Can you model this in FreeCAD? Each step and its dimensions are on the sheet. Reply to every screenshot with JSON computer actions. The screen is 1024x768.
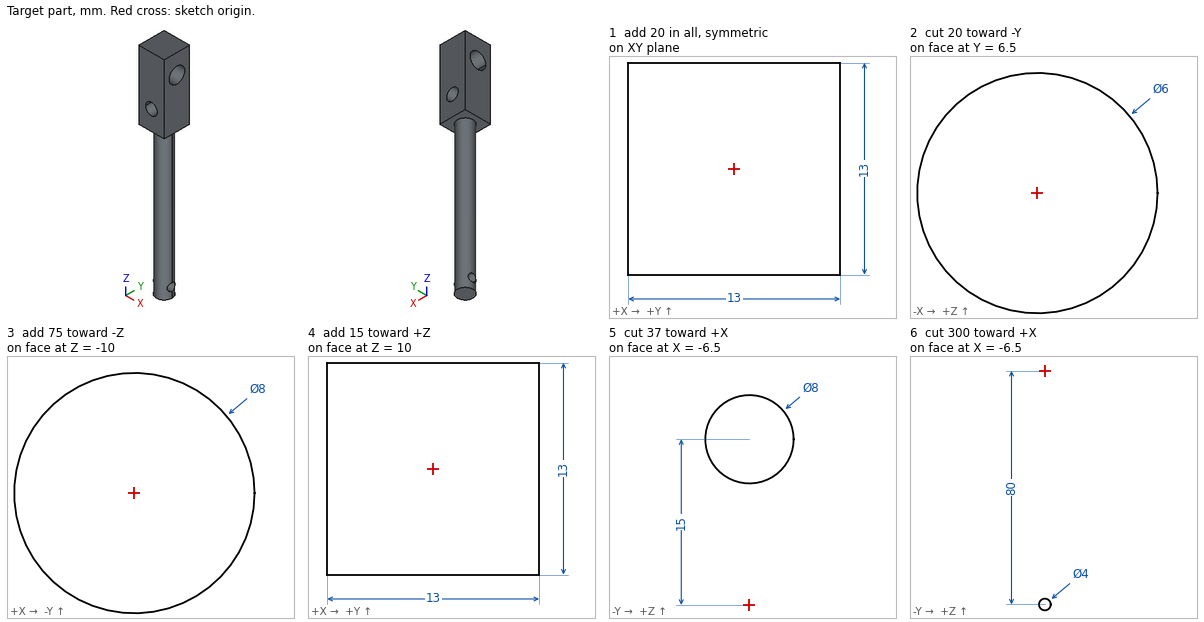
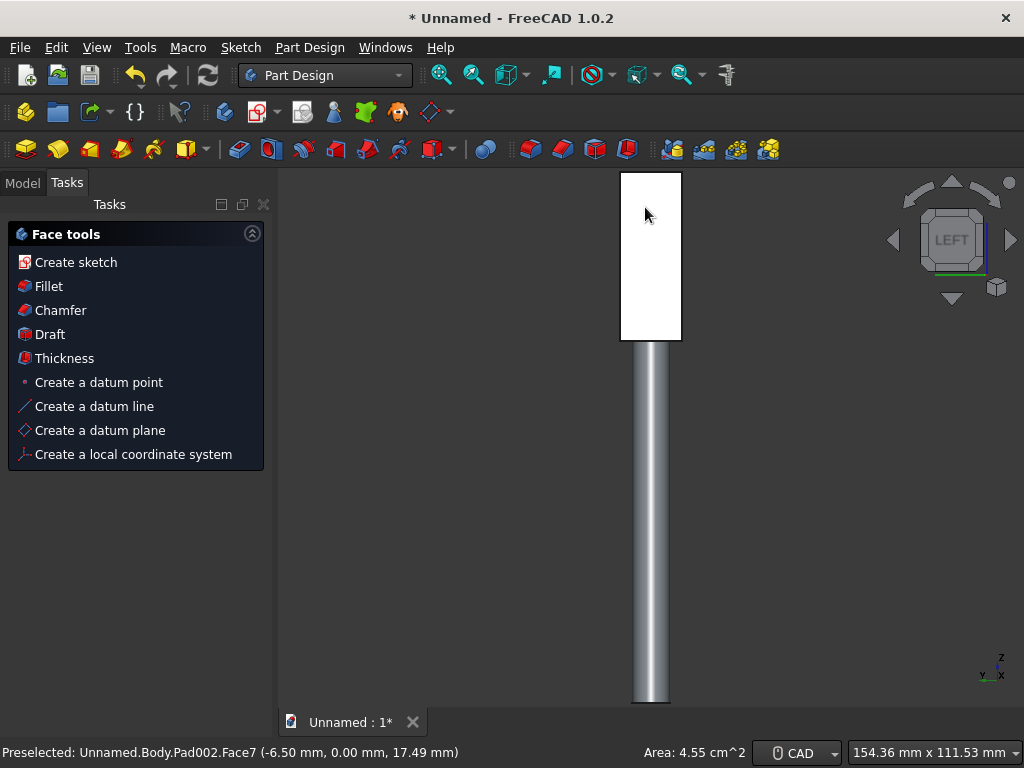
{"action": "left_click", "coordinate": [258, 112]}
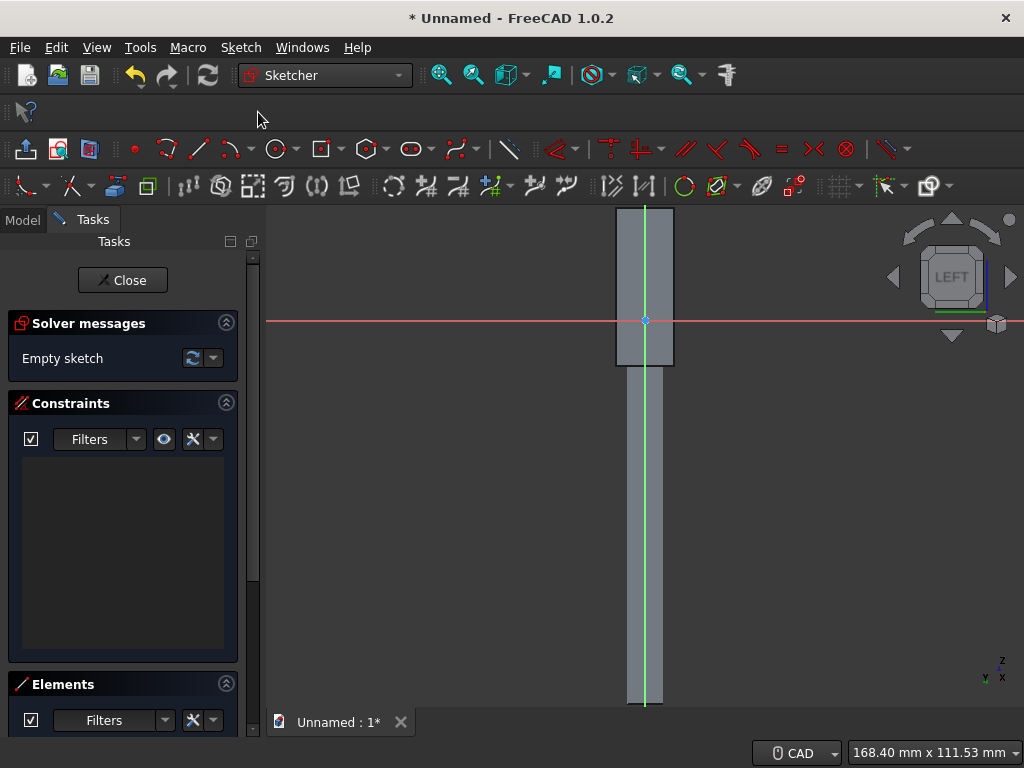
{"action": "scroll", "coordinate": [576, 456], "scroll_direction": "down", "scroll_amount": 5}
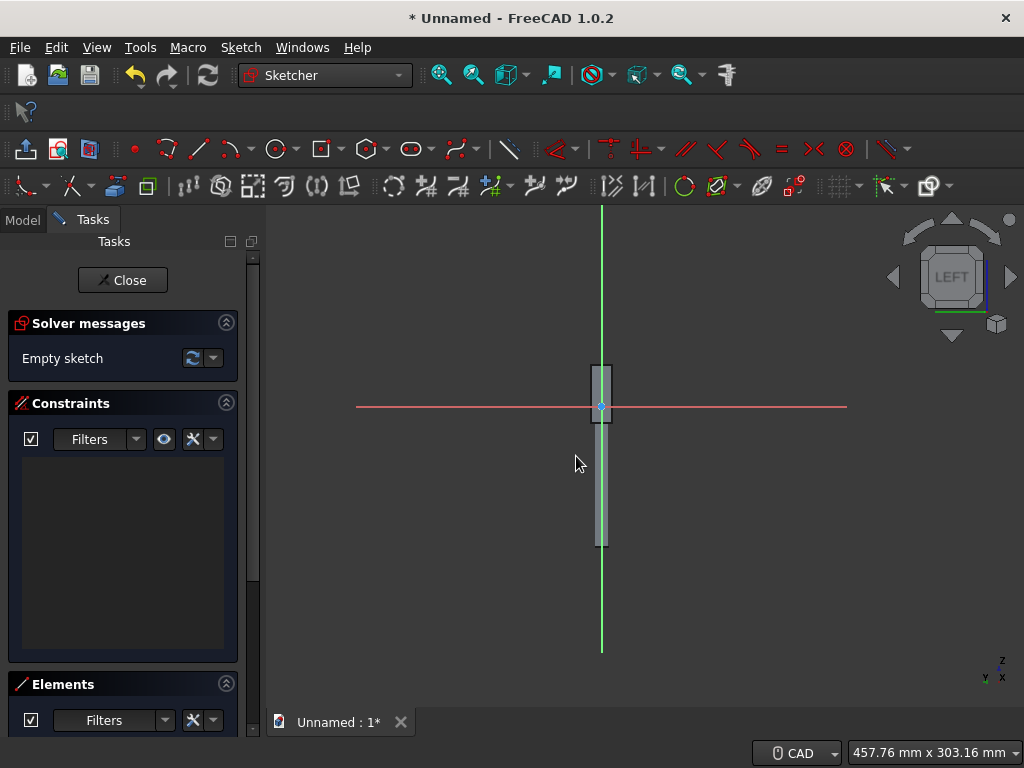
{"action": "scroll", "coordinate": [604, 384], "scroll_direction": "up", "scroll_amount": 12}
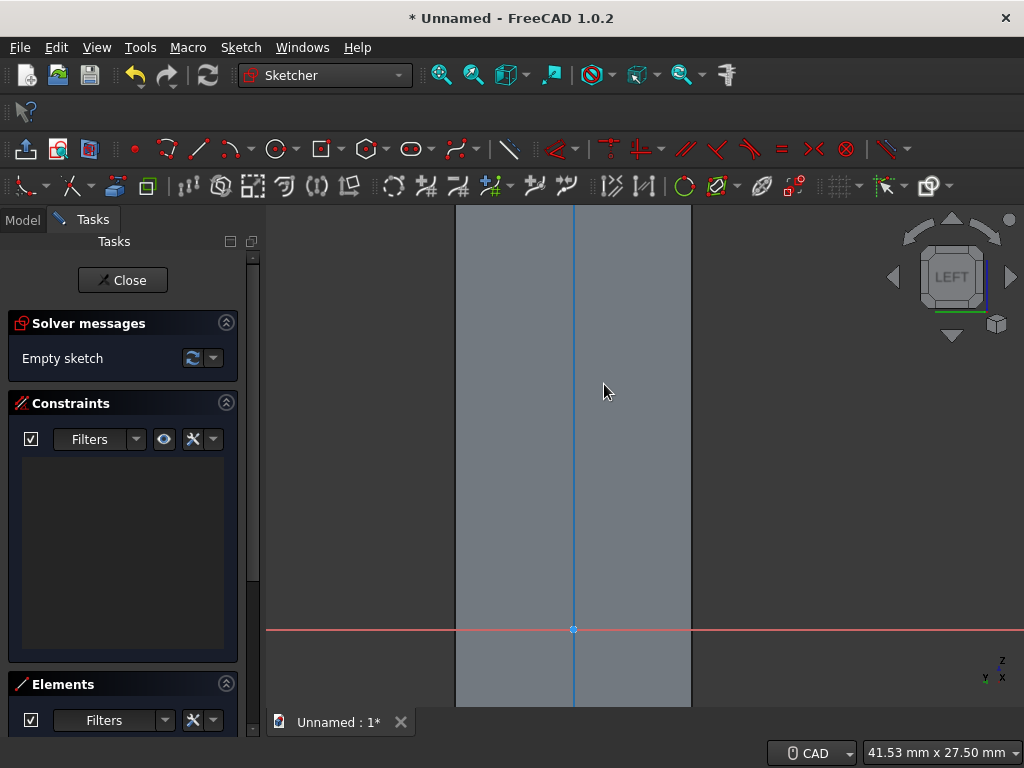
{"action": "left_click", "coordinate": [276, 150]}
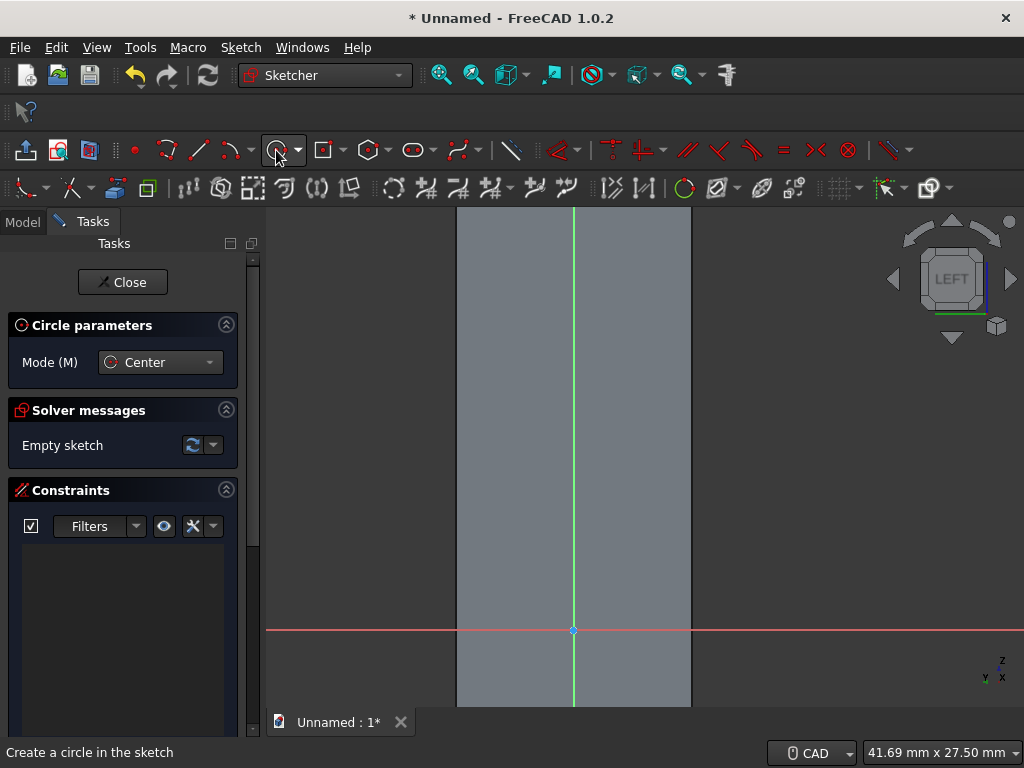
{"action": "left_click", "coordinate": [574, 358]}
{"action": "mouse_move", "coordinate": [625, 306]}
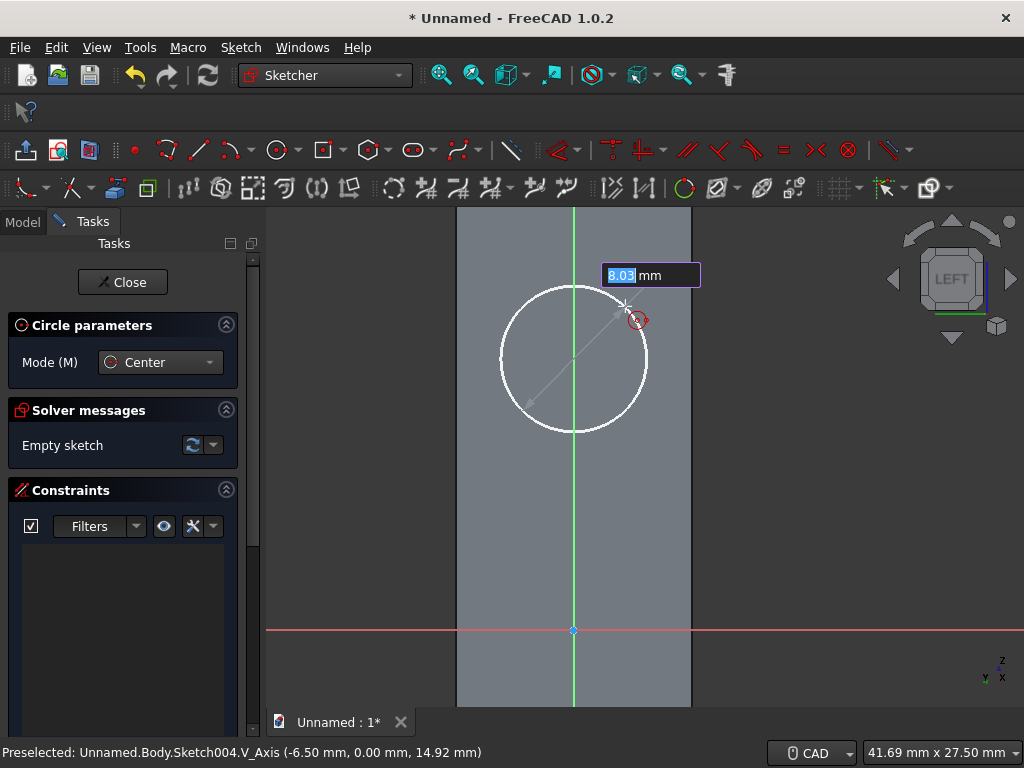
{"action": "type", "text": "8"}
{"action": "key", "text": "Return"}
{"action": "key", "text": "Escape"}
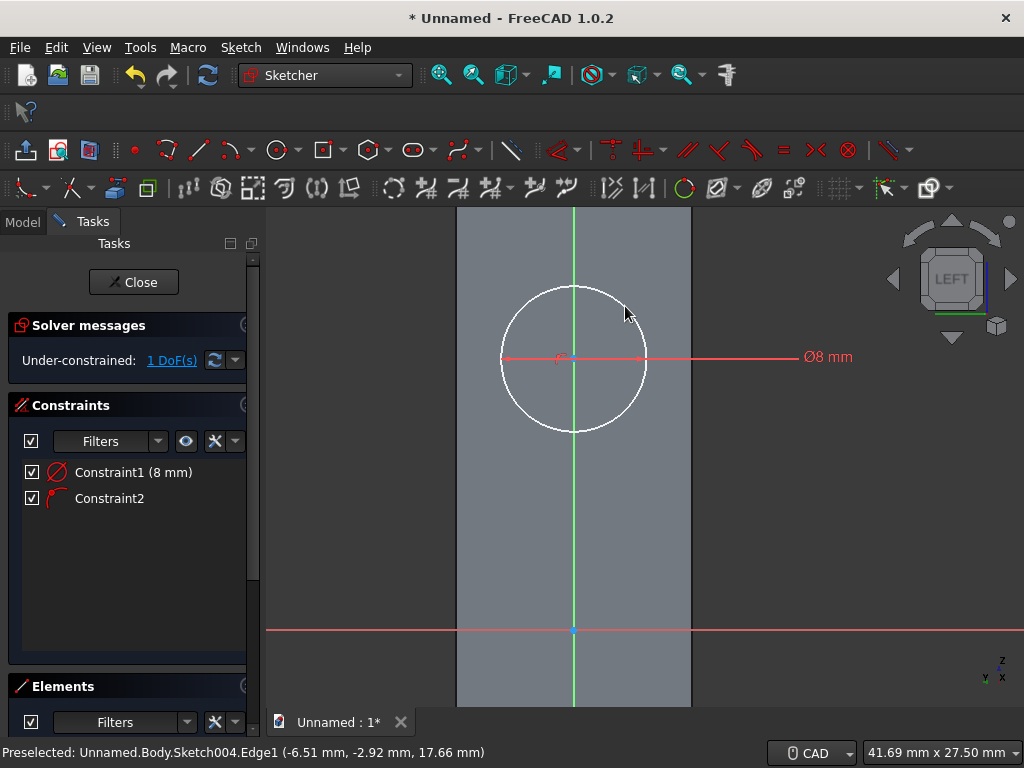
{"action": "left_click", "coordinate": [574, 359]}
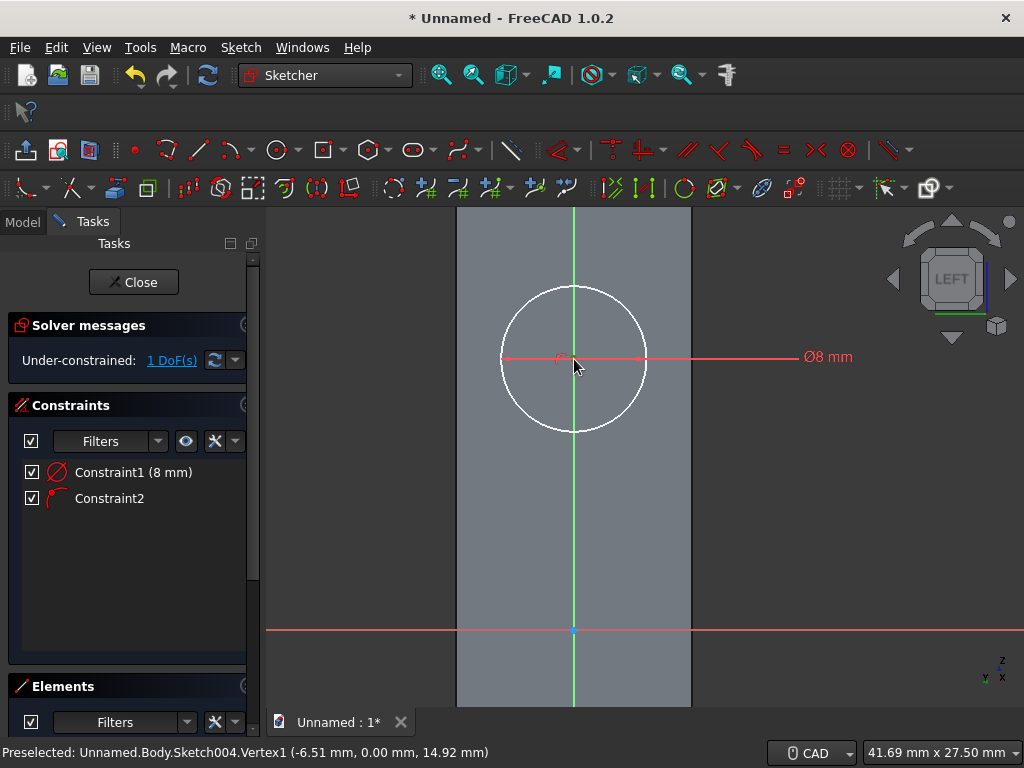
{"action": "key", "text": "i"}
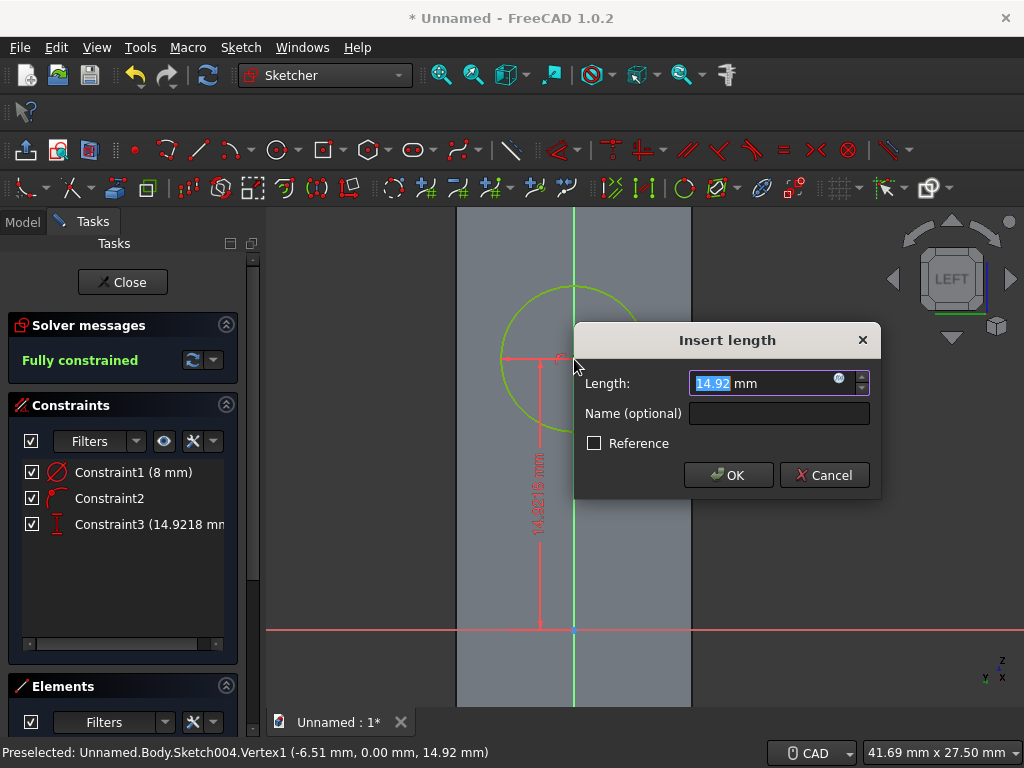
{"action": "type", "text": "15"}
{"action": "key", "text": "Return"}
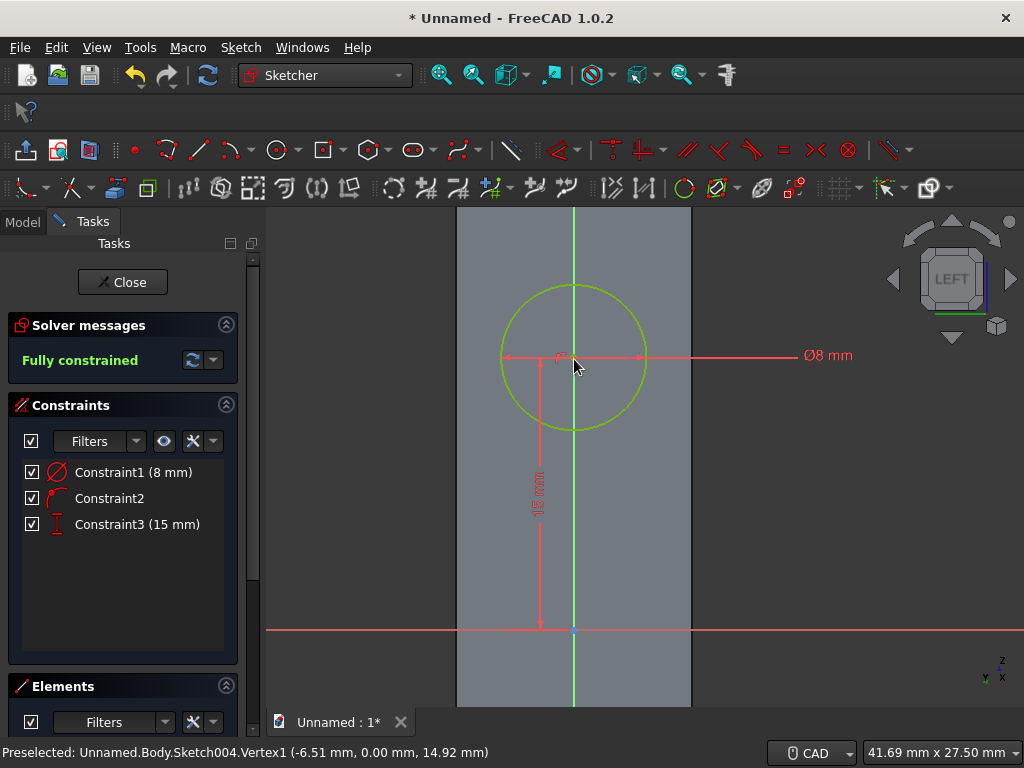
{"action": "left_click", "coordinate": [123, 282]}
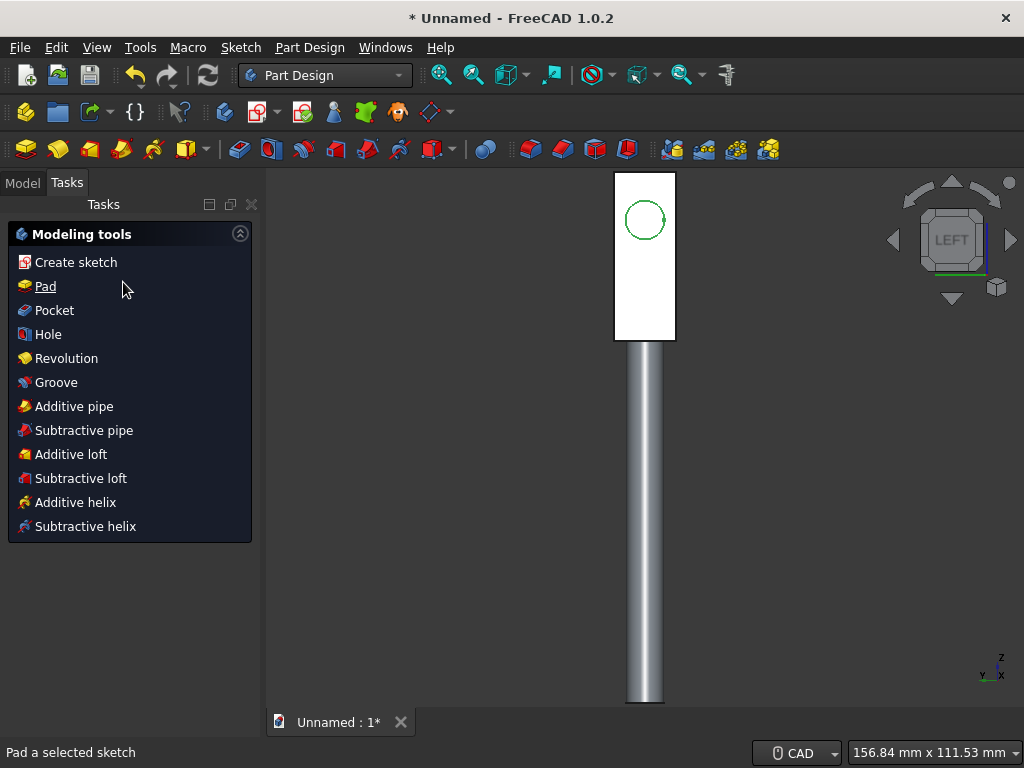
{"action": "left_click", "coordinate": [240, 150]}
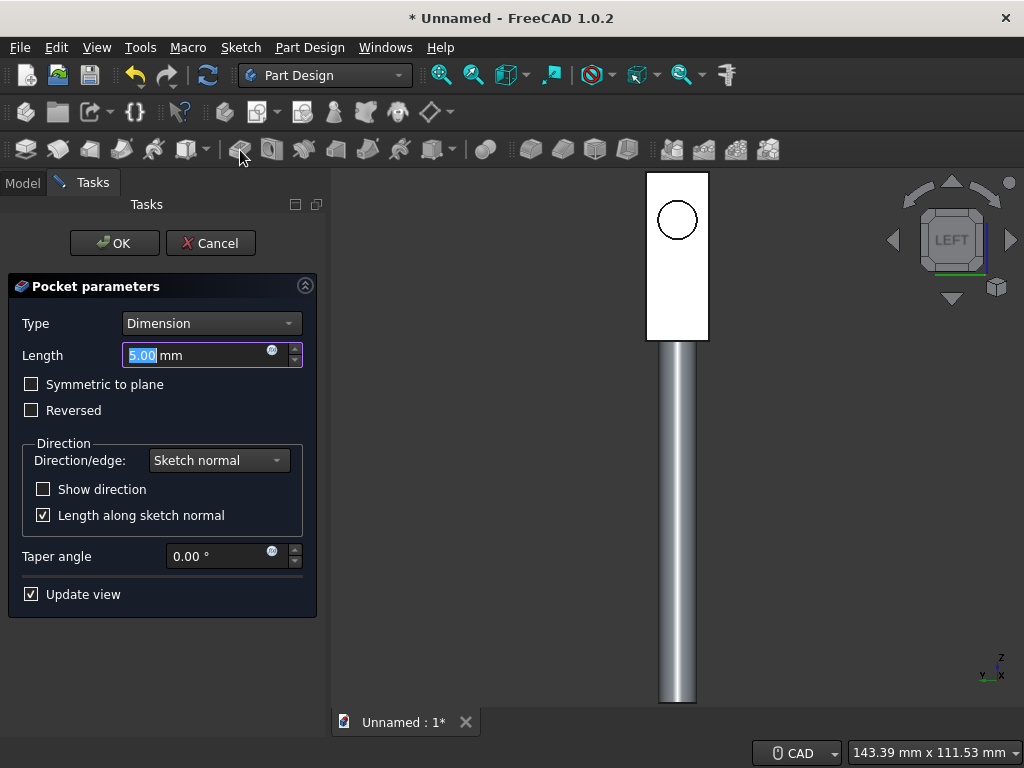
{"action": "type", "text": "37"}
{"action": "key", "text": "Tab"}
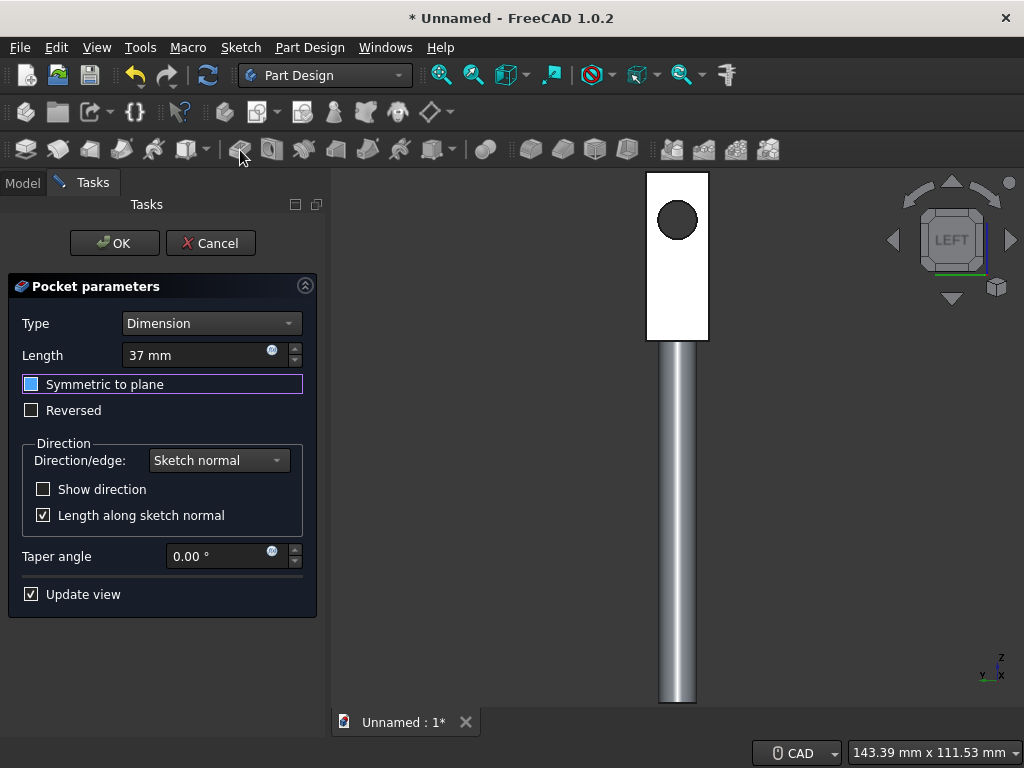
{"action": "left_click", "coordinate": [115, 243]}